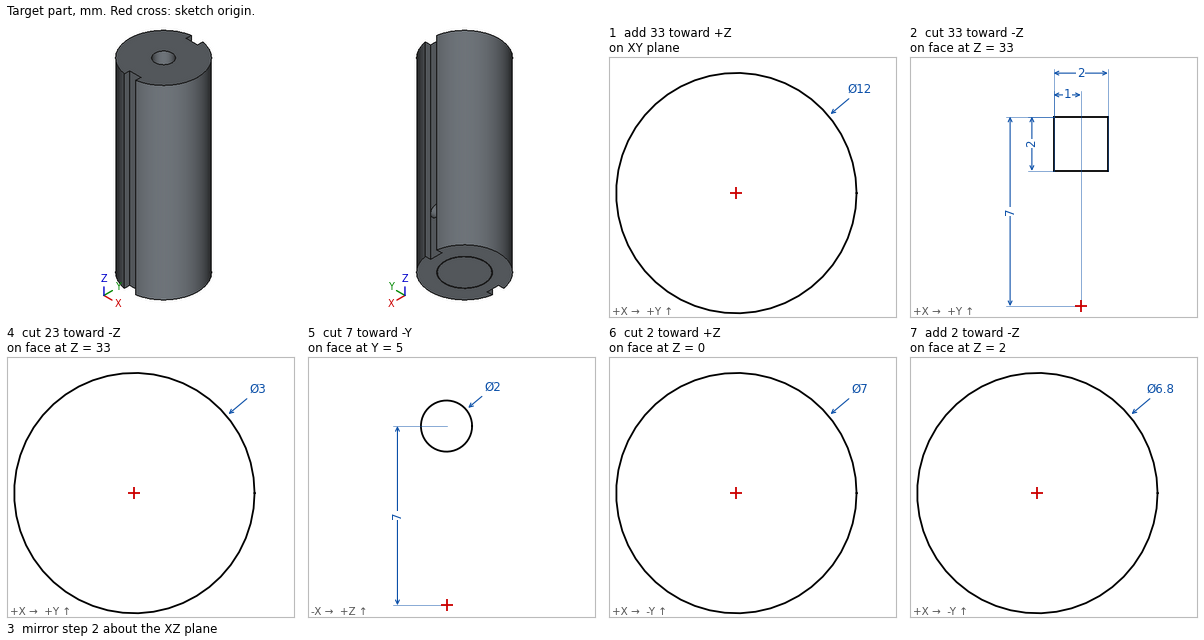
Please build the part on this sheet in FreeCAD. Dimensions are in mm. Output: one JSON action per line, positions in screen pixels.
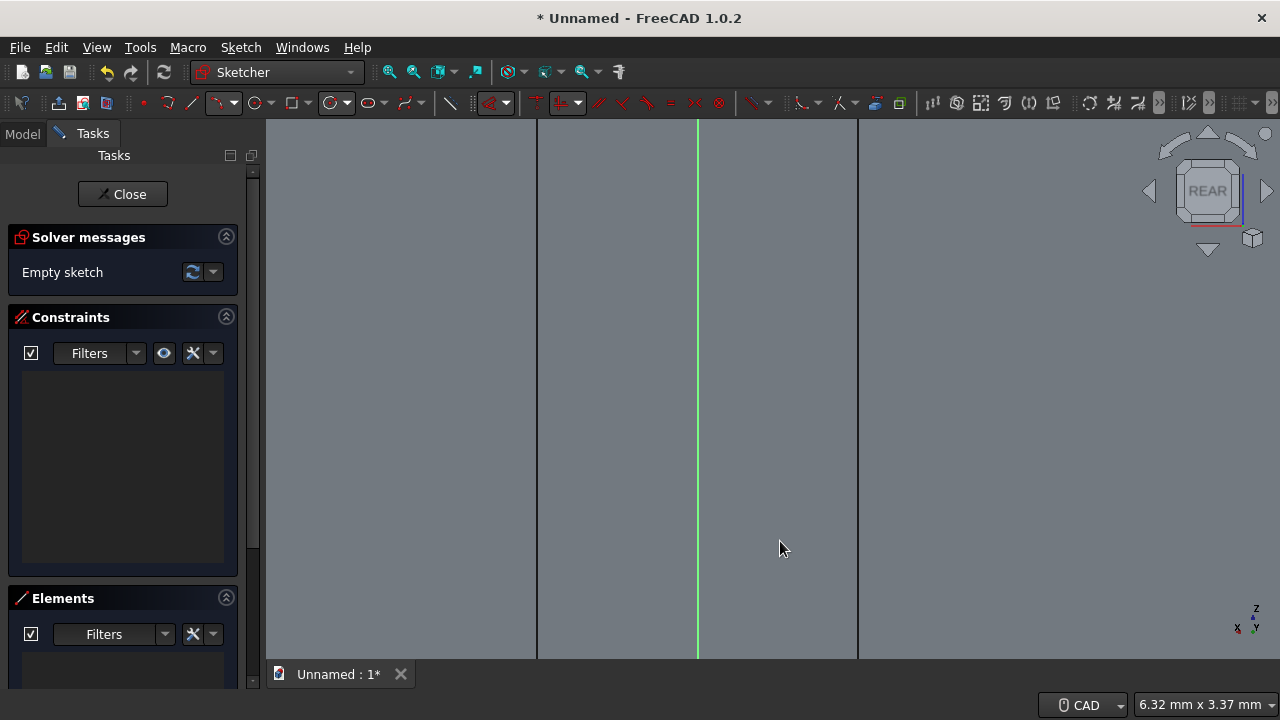
{"action": "key", "text": "g c"}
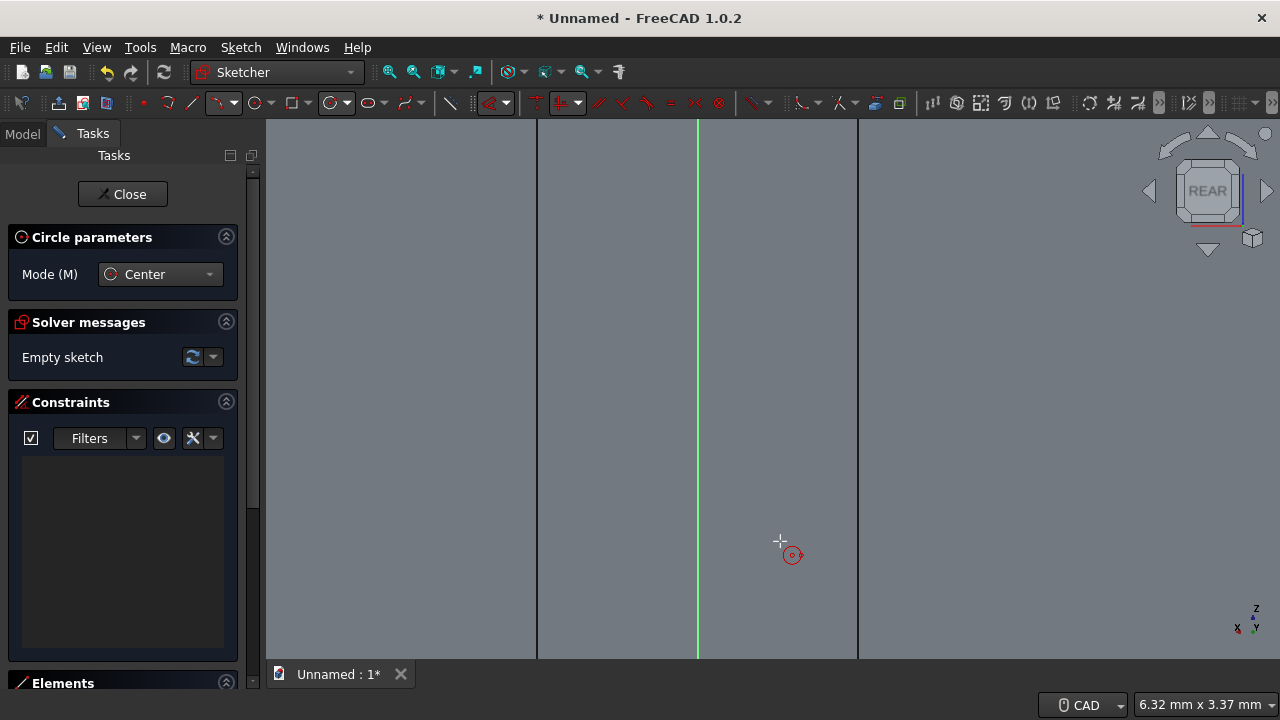
{"action": "left_click", "coordinate": [698, 382]}
{"action": "left_click", "coordinate": [811, 268]}
{"action": "key", "text": "Escape"}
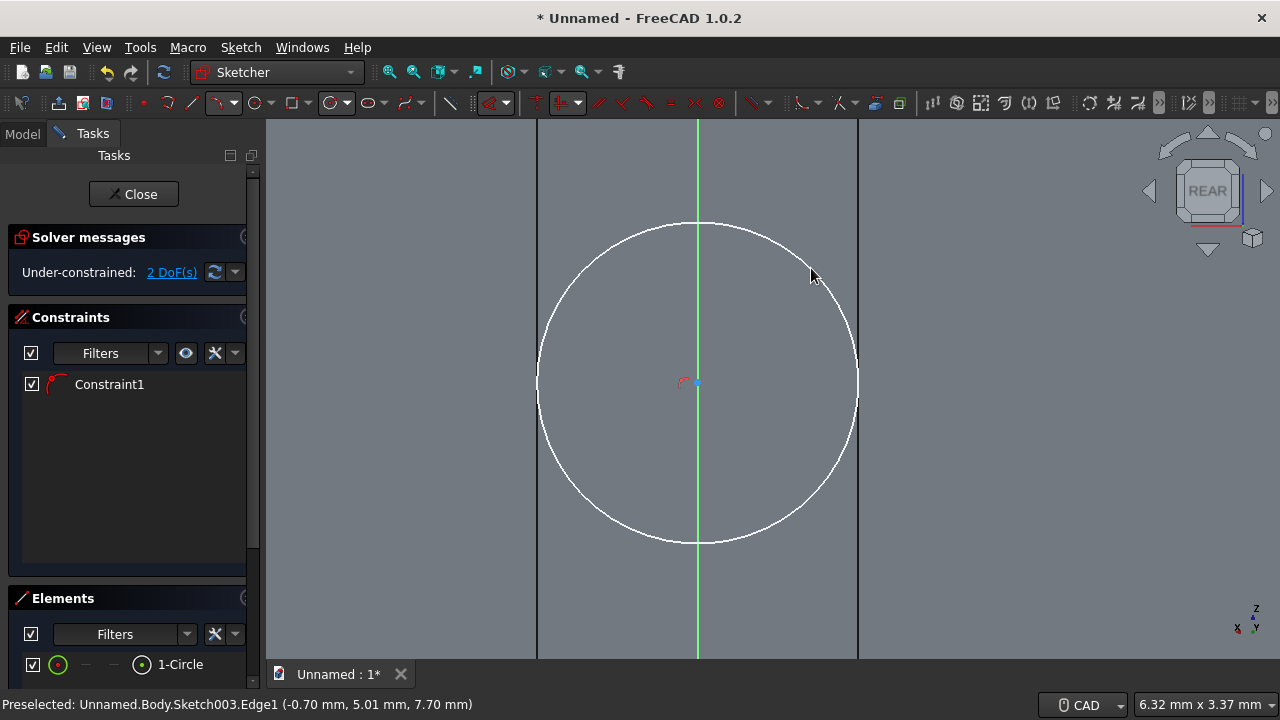
{"action": "key", "text": "d"}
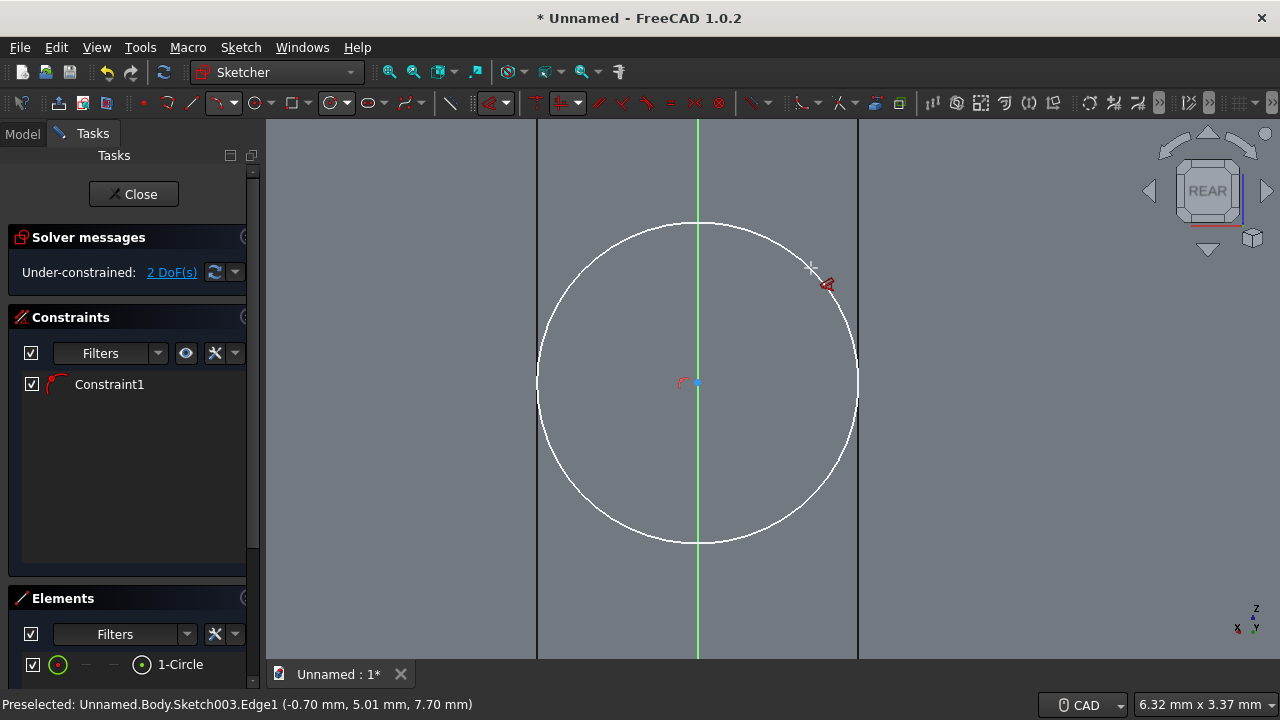
{"action": "left_click", "coordinate": [811, 269]}
{"action": "left_click", "coordinate": [834, 246]}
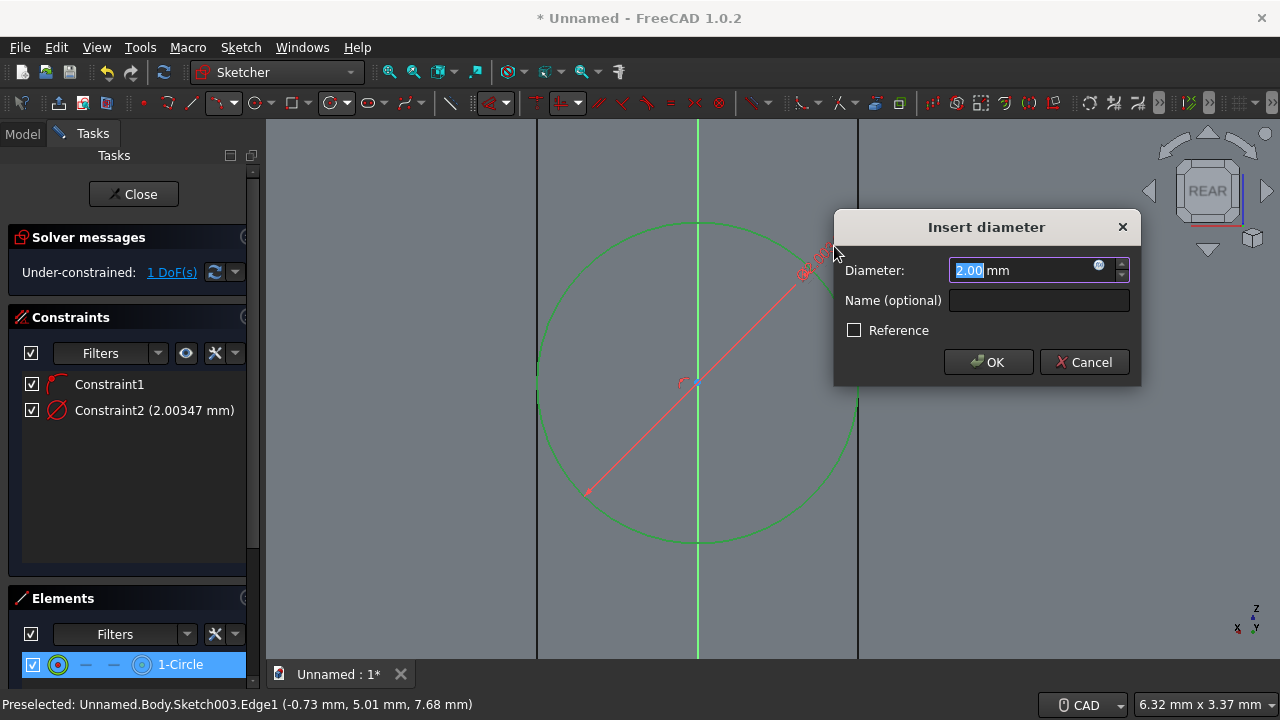
{"action": "type", "text": "2"}
{"action": "key", "text": "Return"}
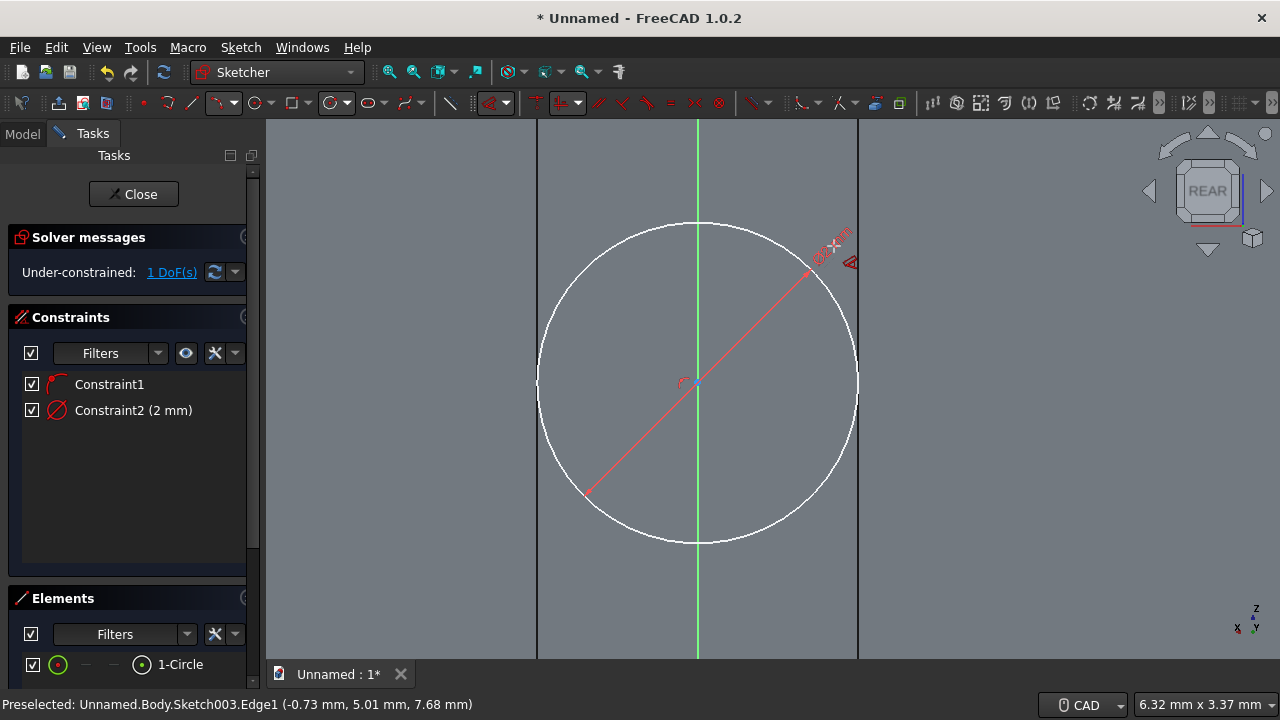
{"action": "left_click", "coordinate": [698, 383]}
{"action": "left_click", "coordinate": [732, 507]}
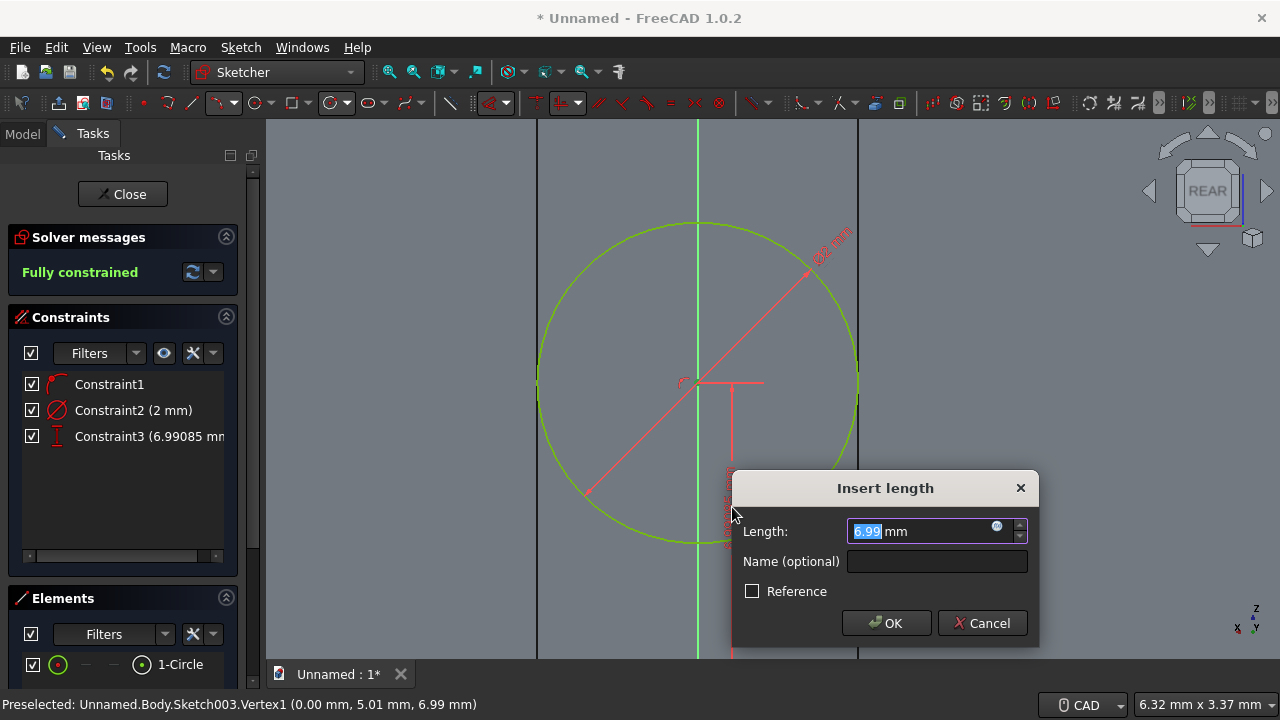
{"action": "type", "text": "7"}
{"action": "key", "text": "Return"}
{"action": "key", "text": "Escape"}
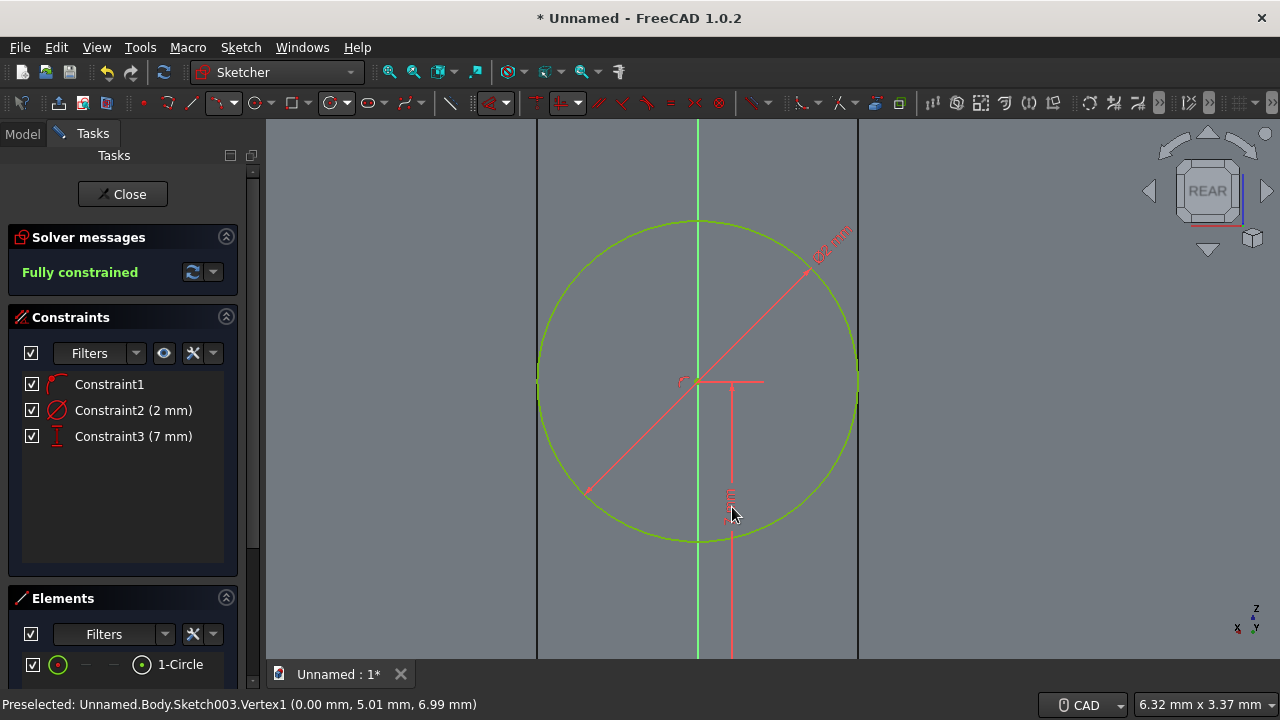
{"action": "left_click", "coordinate": [123, 194]}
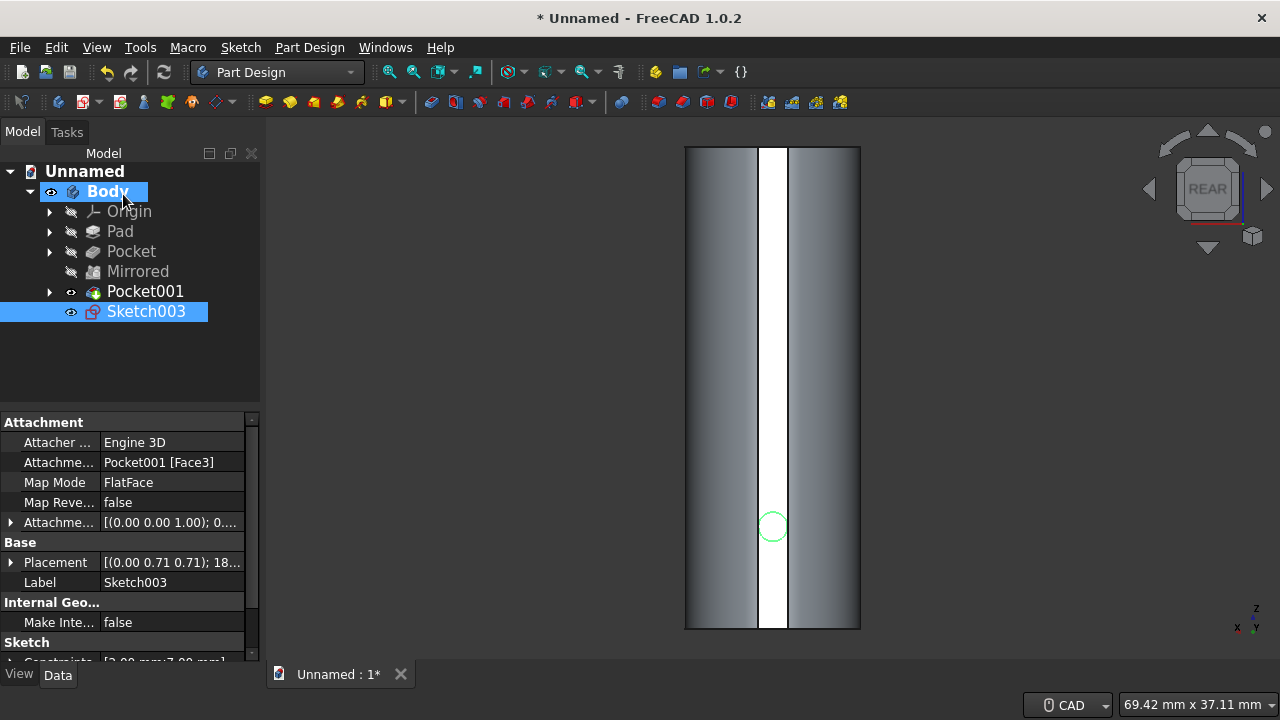
{"action": "left_click", "coordinate": [432, 102]}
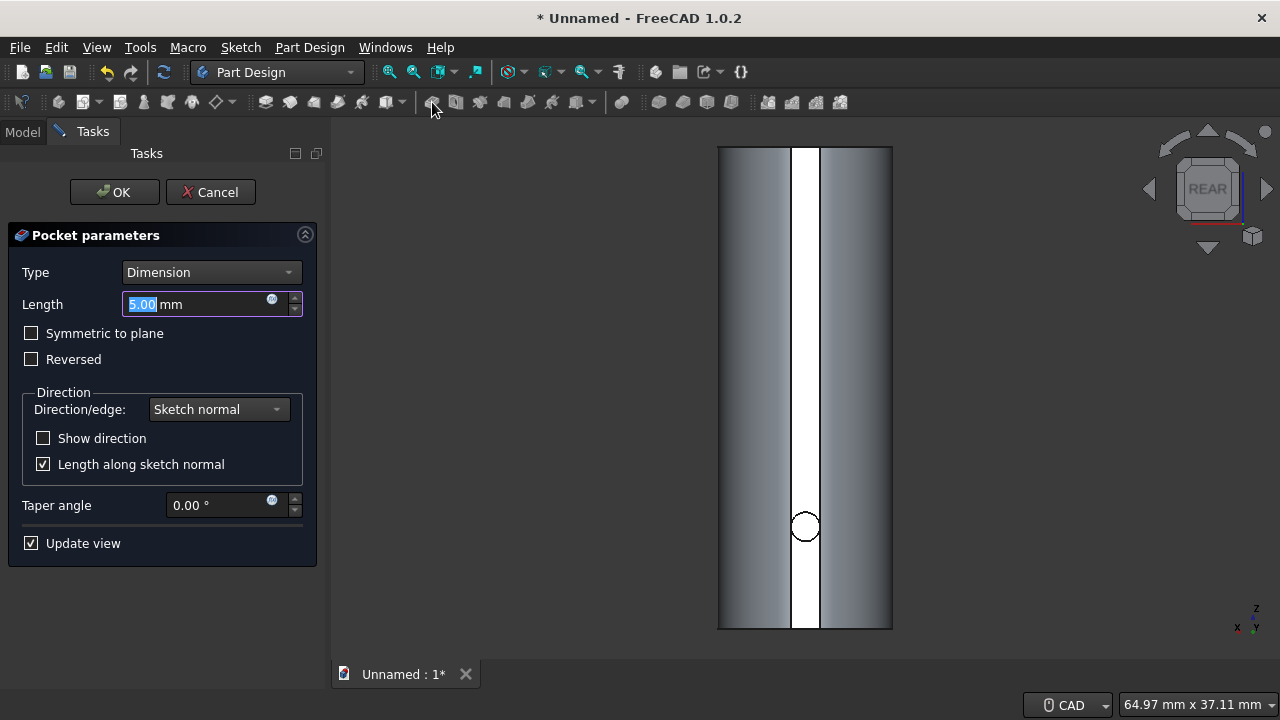
{"action": "type", "text": "7"}
{"action": "key", "text": "Tab"}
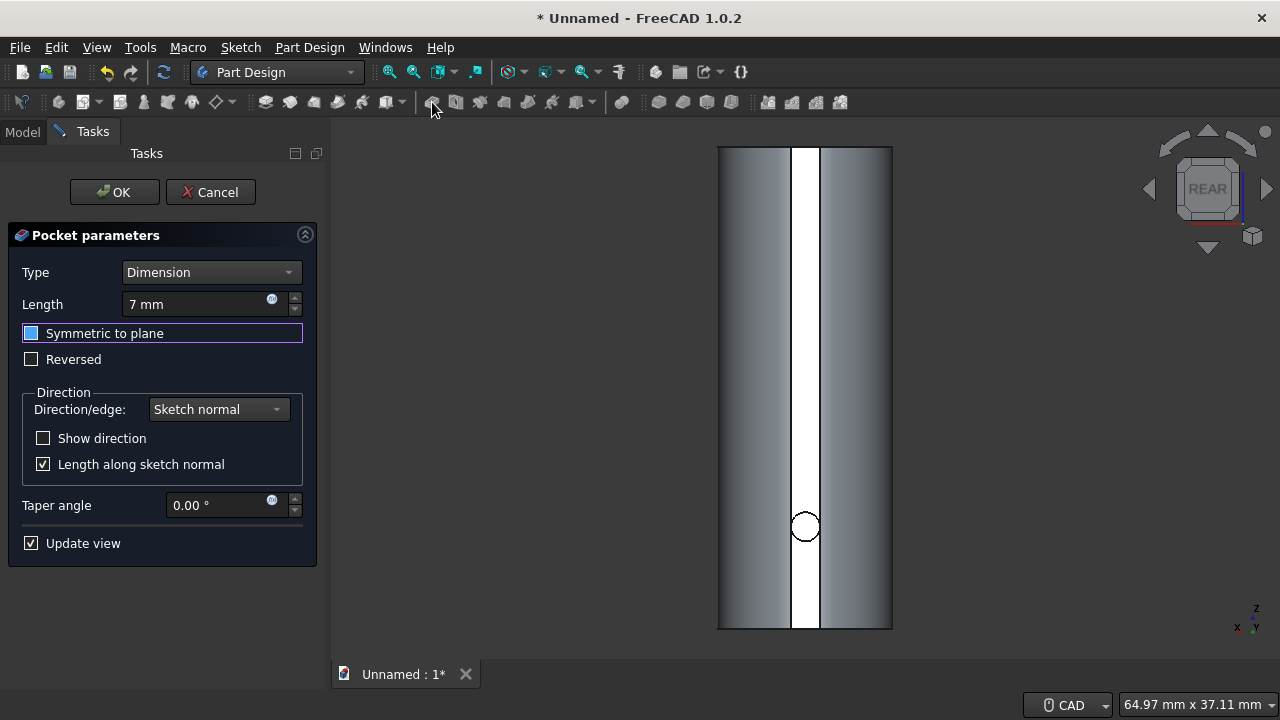
{"action": "left_click", "coordinate": [115, 192]}